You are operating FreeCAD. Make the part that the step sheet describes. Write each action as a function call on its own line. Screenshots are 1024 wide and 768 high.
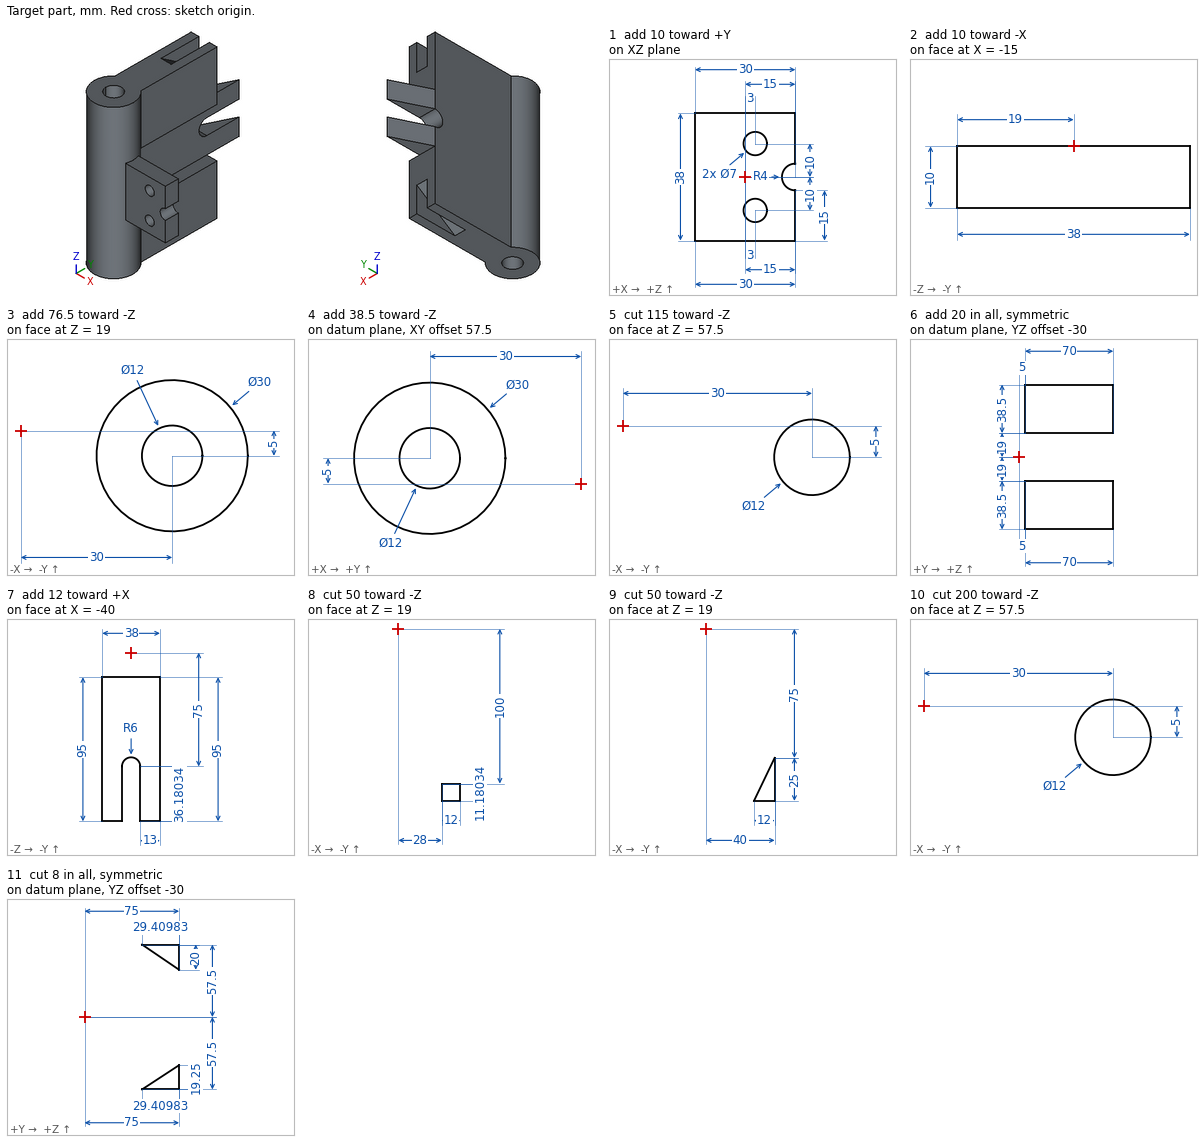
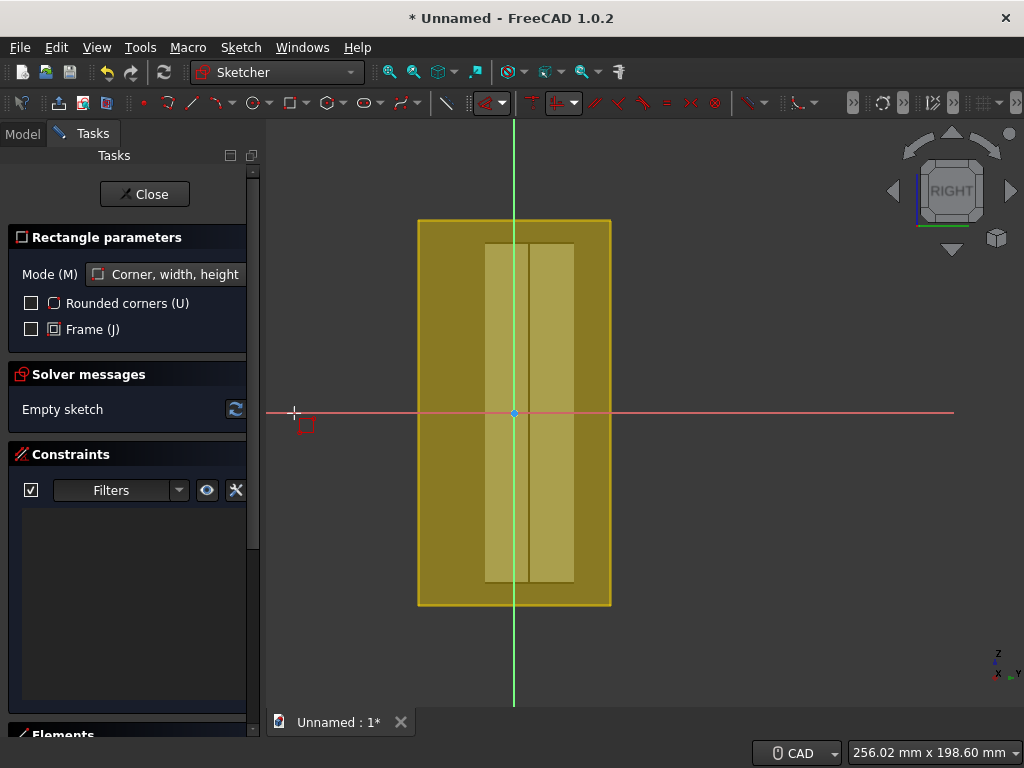
click(529, 469)
click(737, 583)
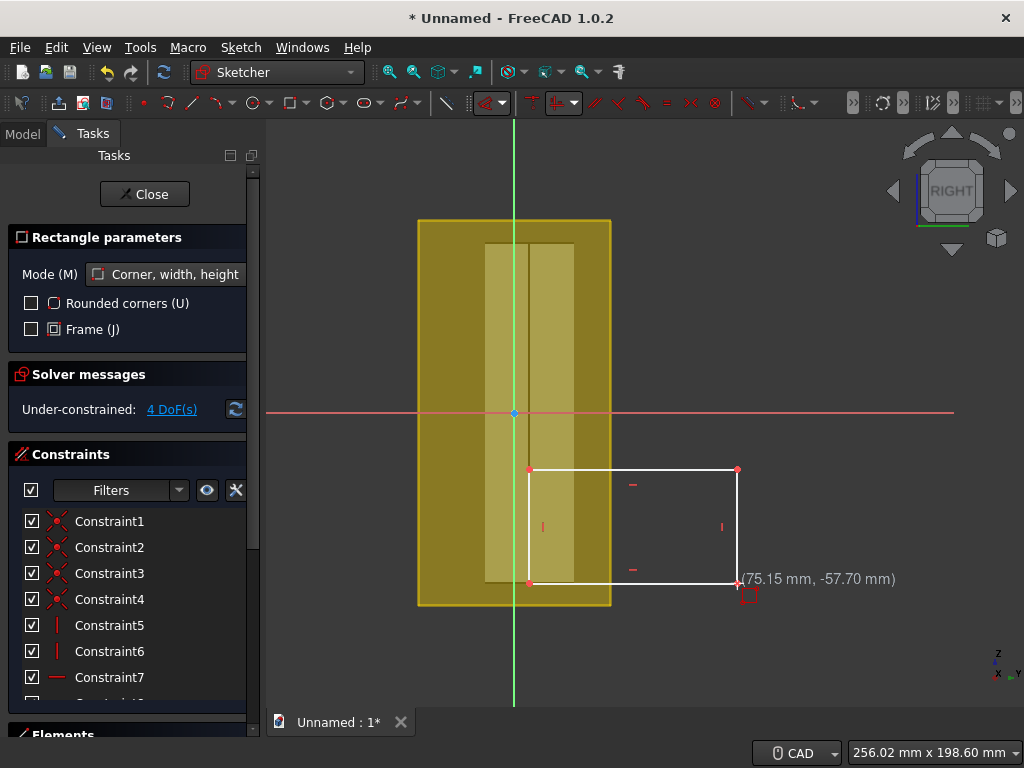
click(529, 243)
click(737, 357)
key(Escape)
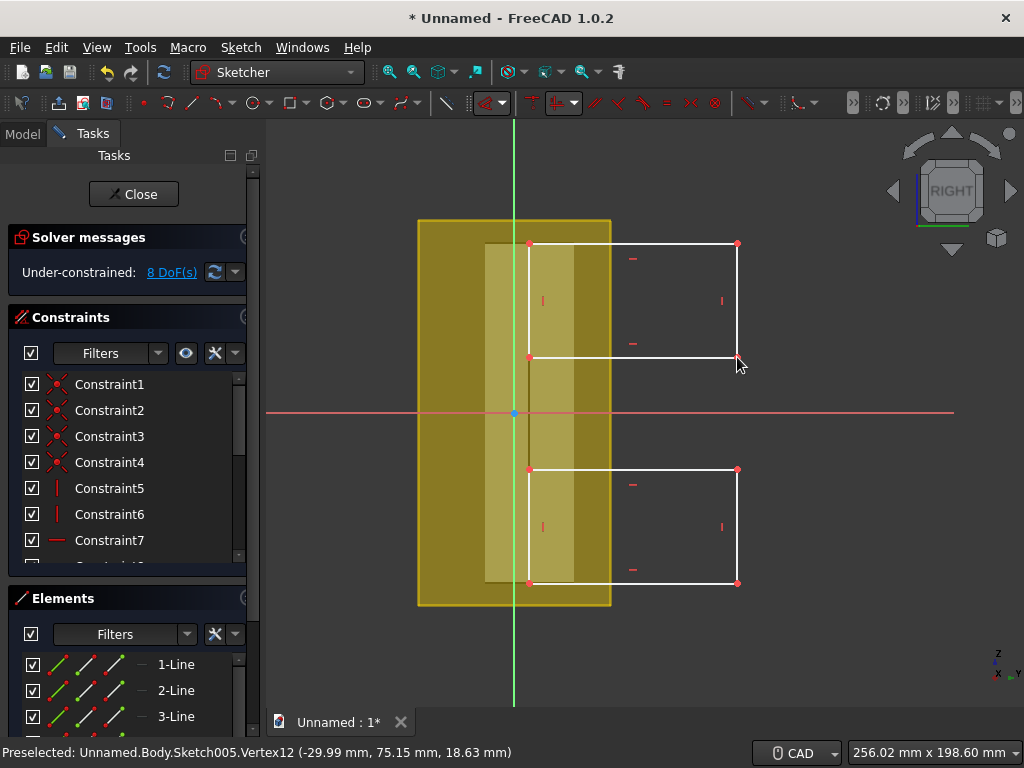
click(591, 584)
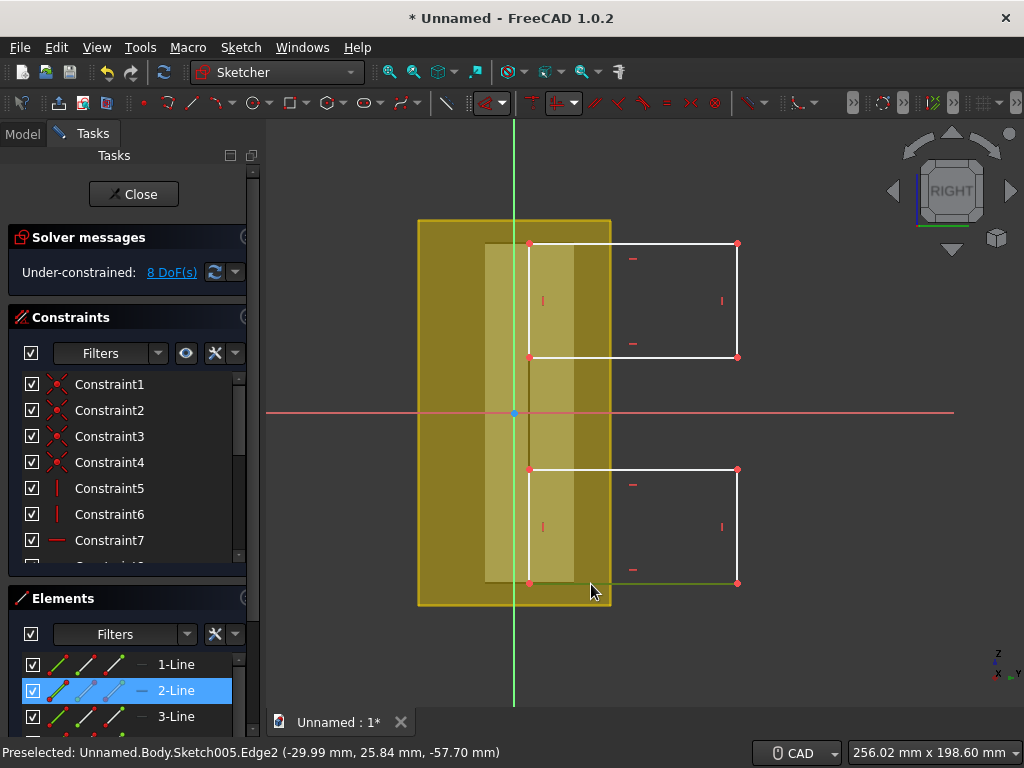
click(504, 104)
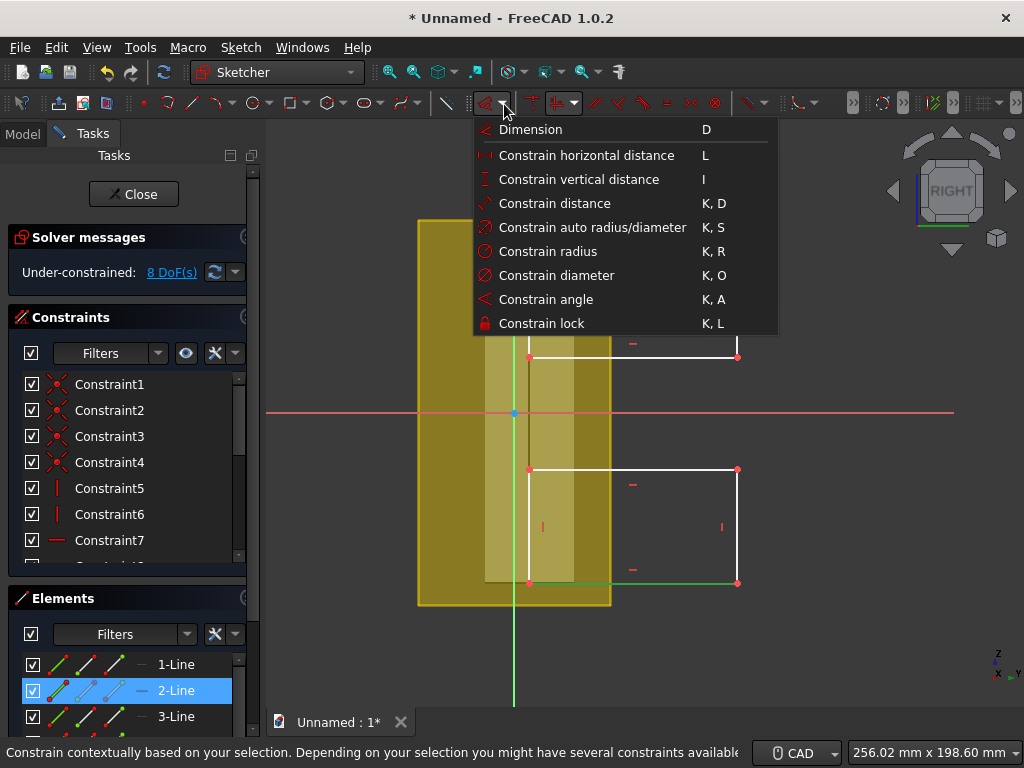
click(626, 155)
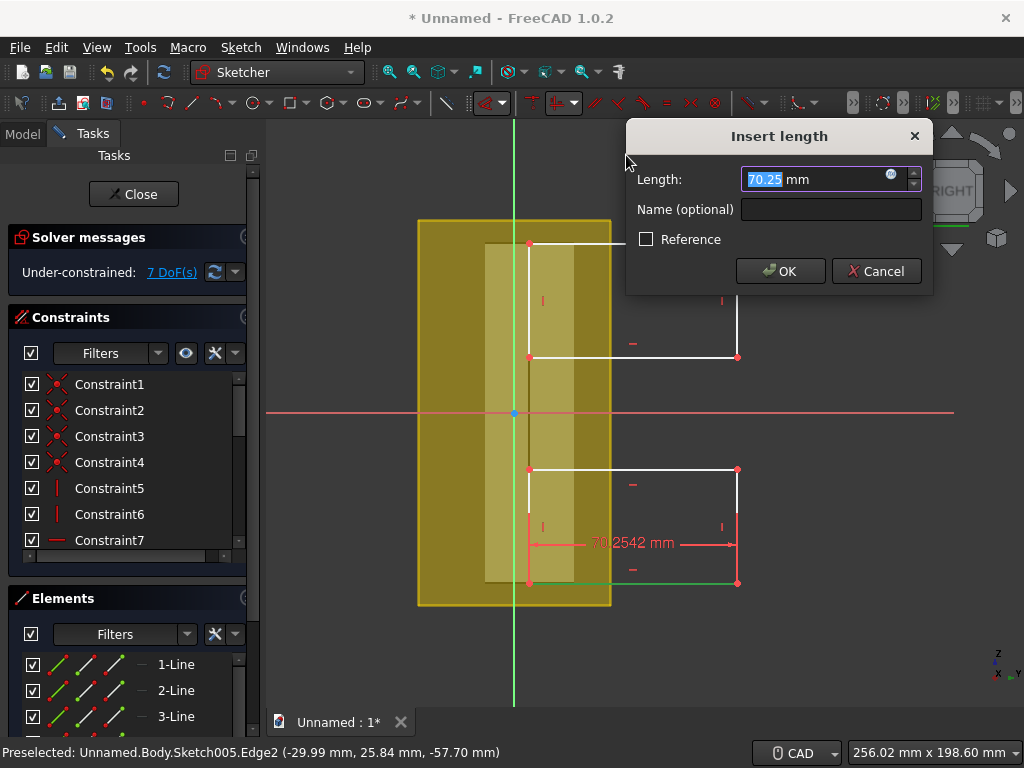
text(70)
key(Return)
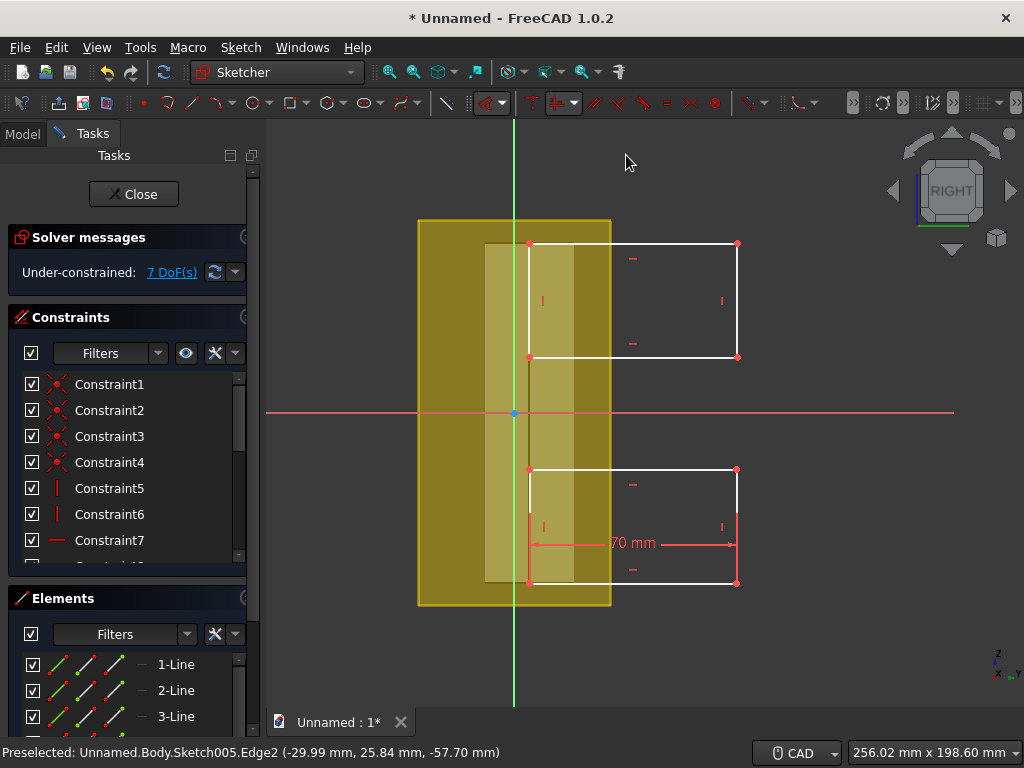
click(591, 358)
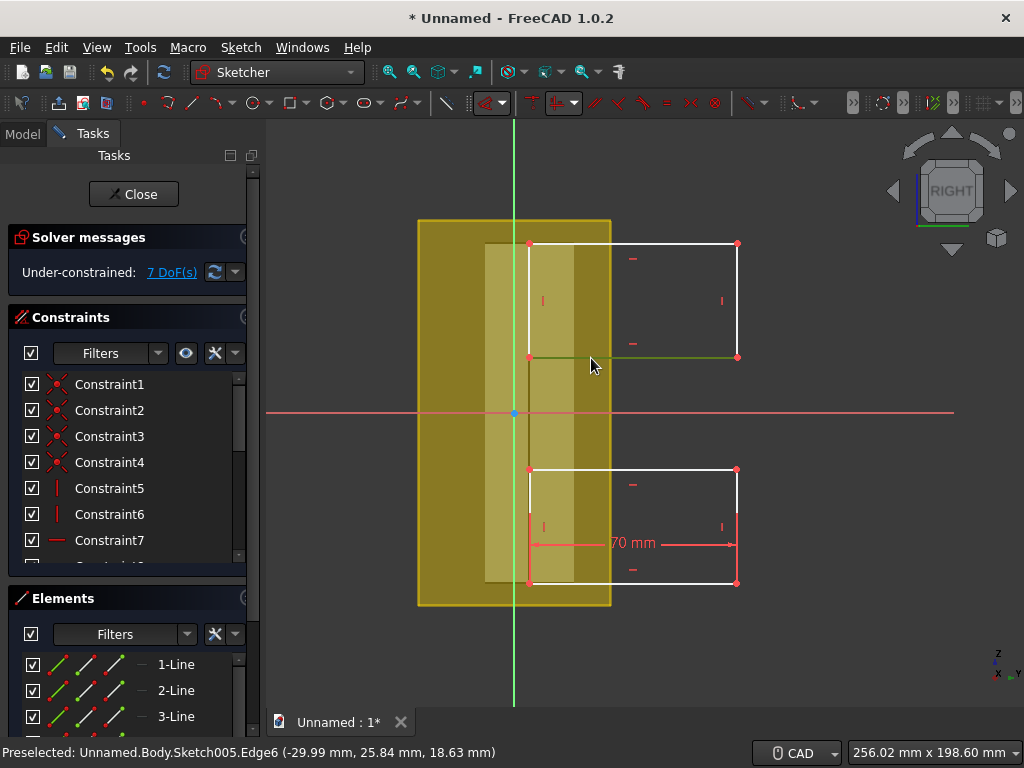
key(l)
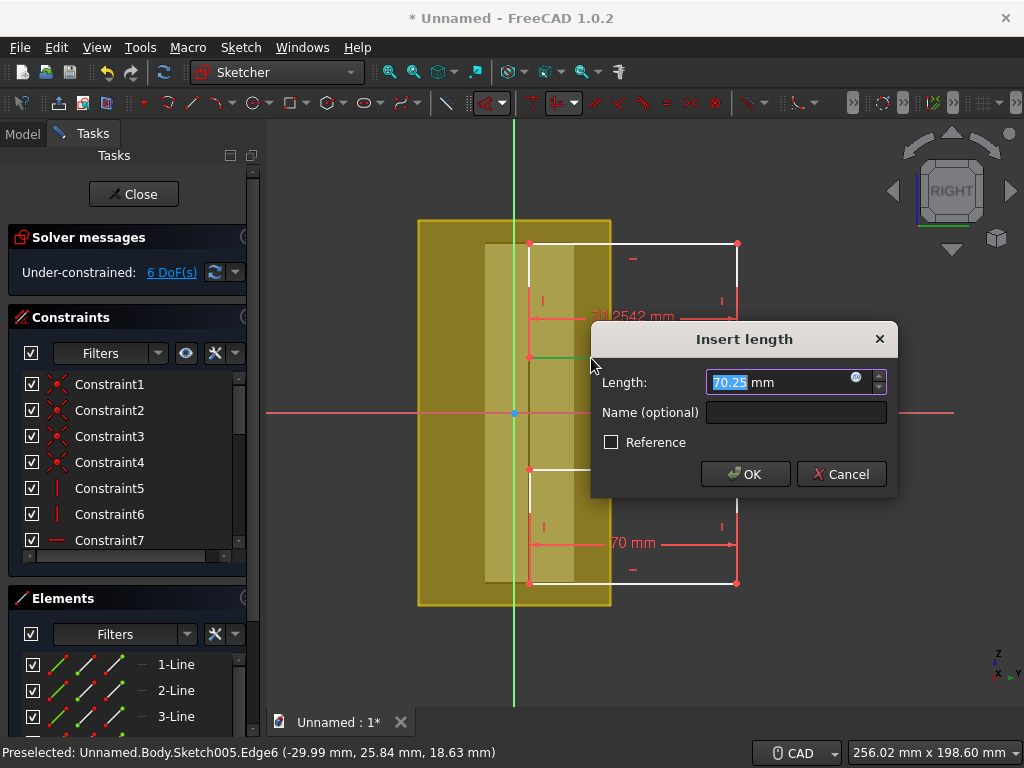
text(70)
key(Return)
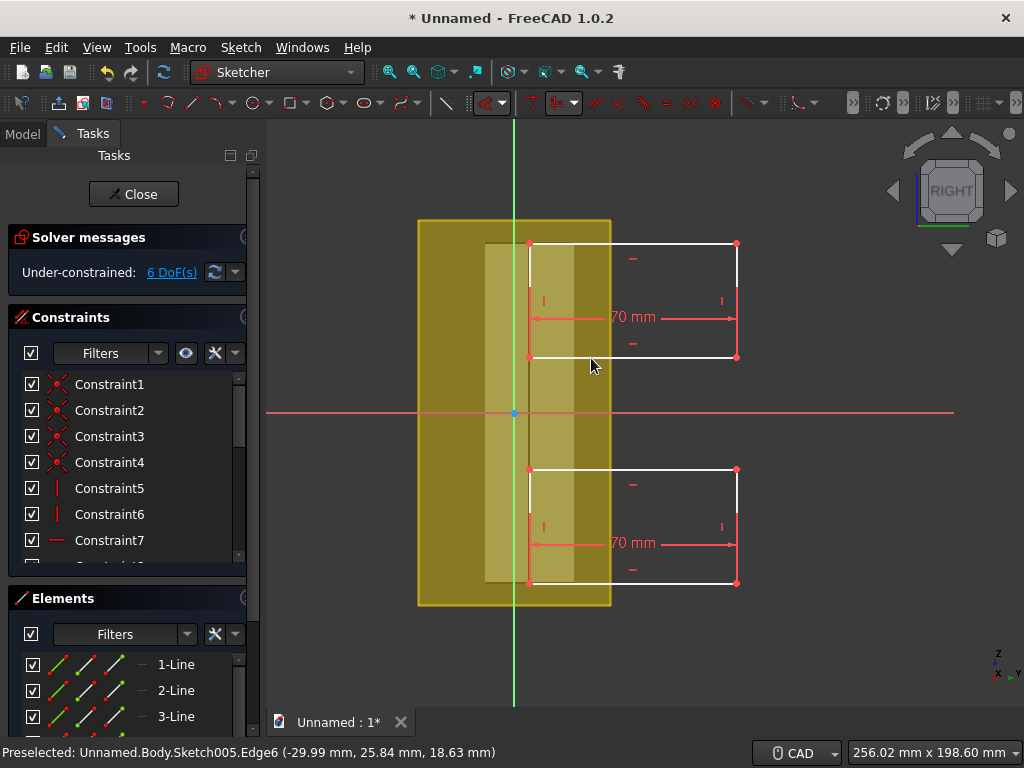
scroll(530, 470, up, 5)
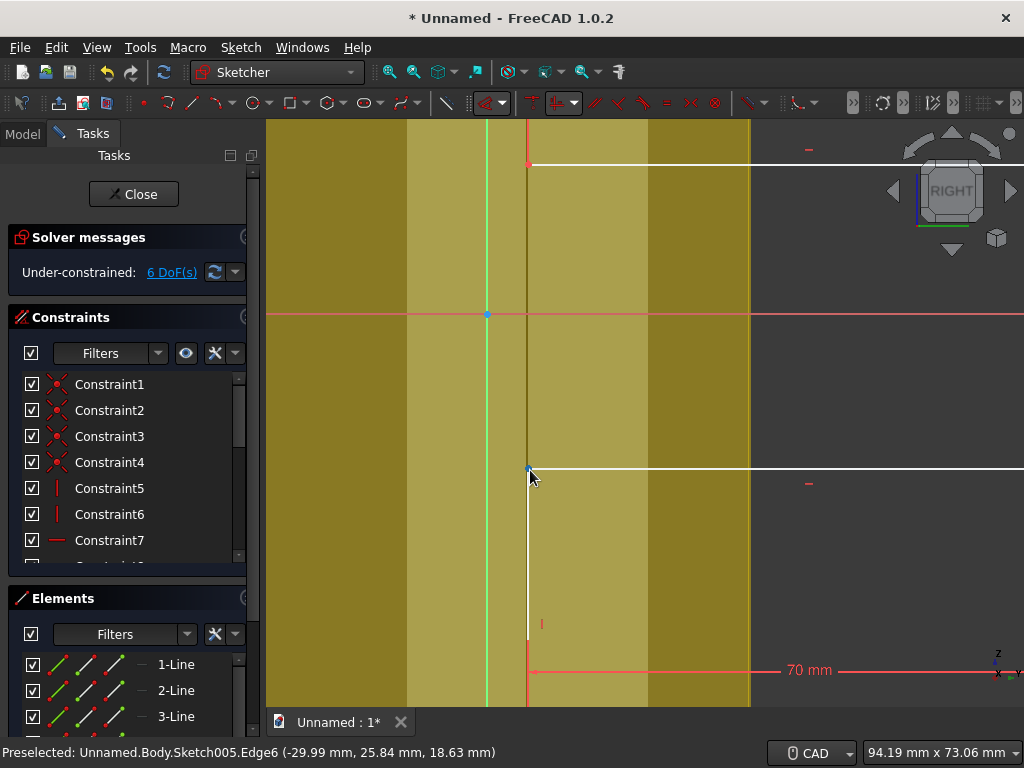
click(528, 469)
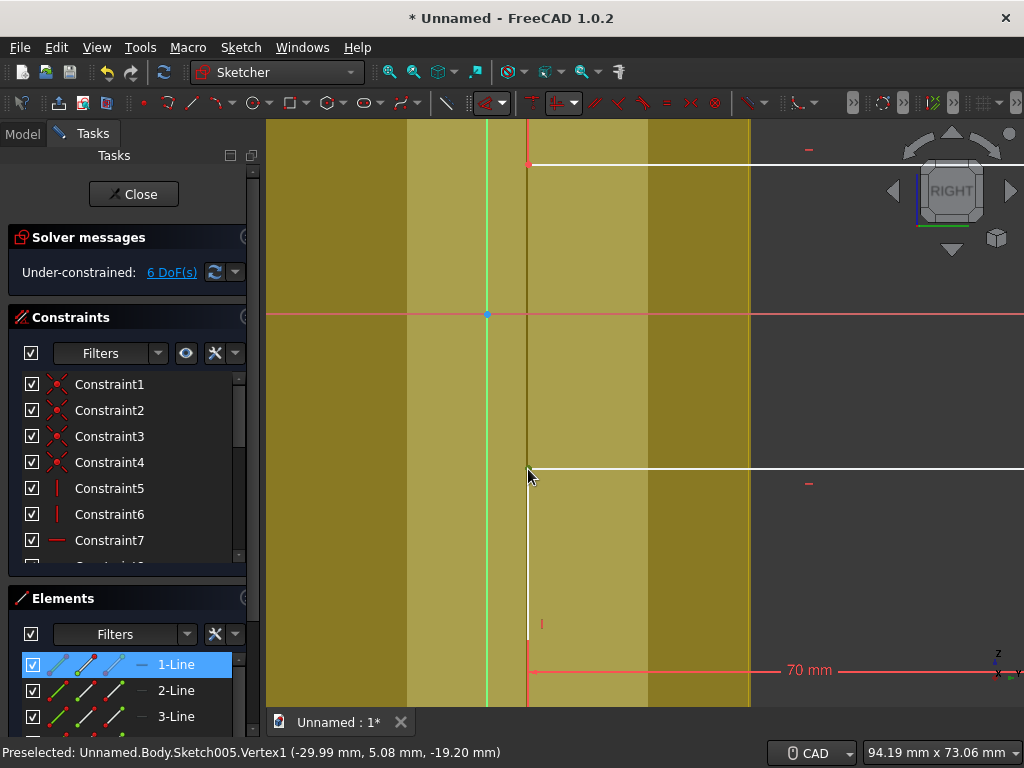
click(504, 104)